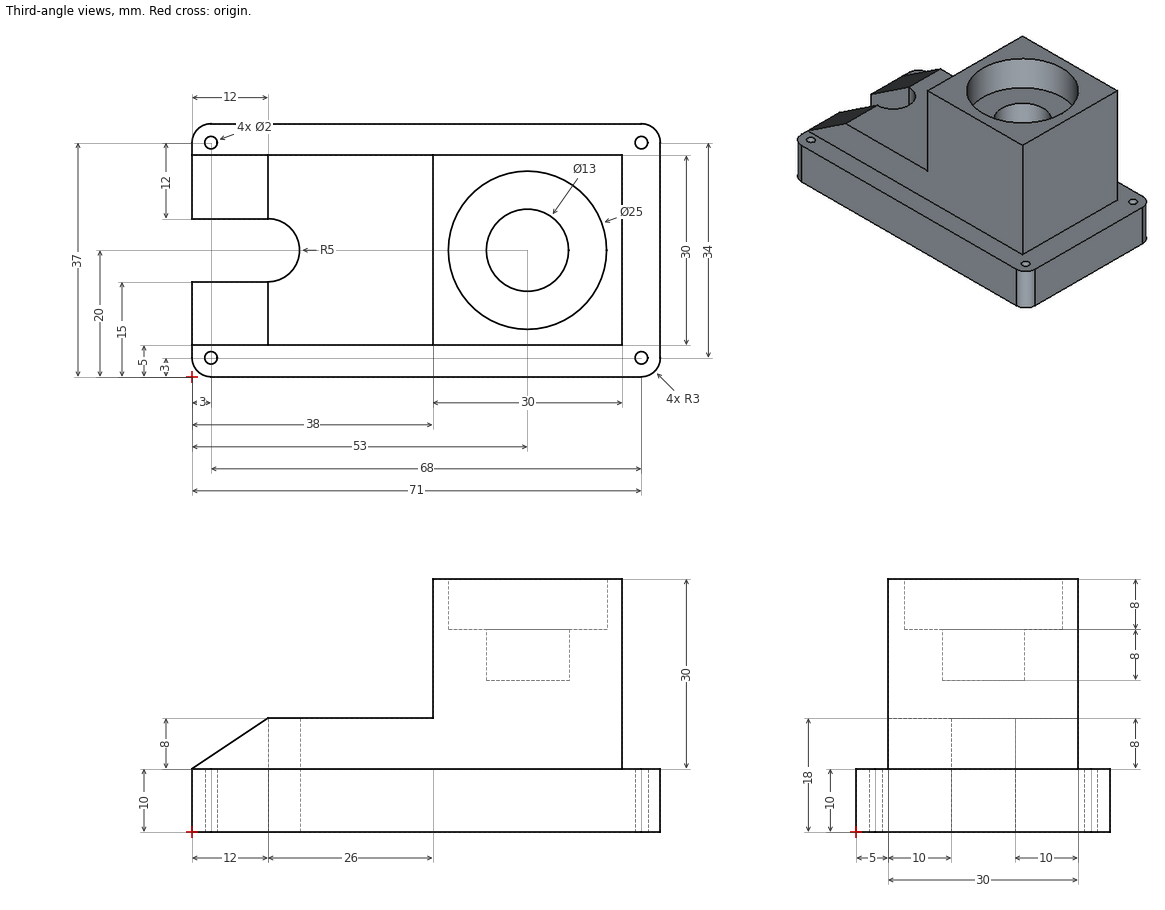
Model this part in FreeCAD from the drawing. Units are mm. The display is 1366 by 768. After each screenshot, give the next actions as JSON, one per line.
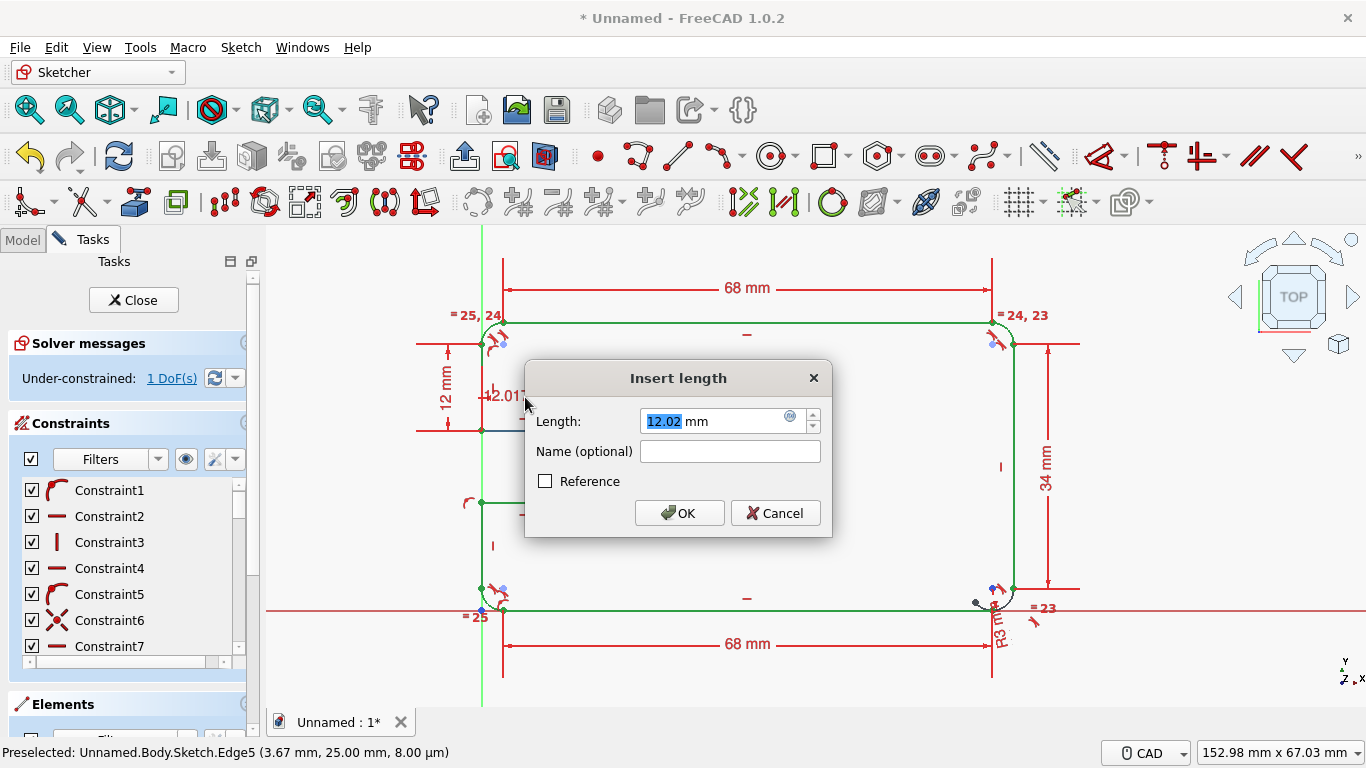
{"action": "type", "text": "12"}
{"action": "key", "text": "Return"}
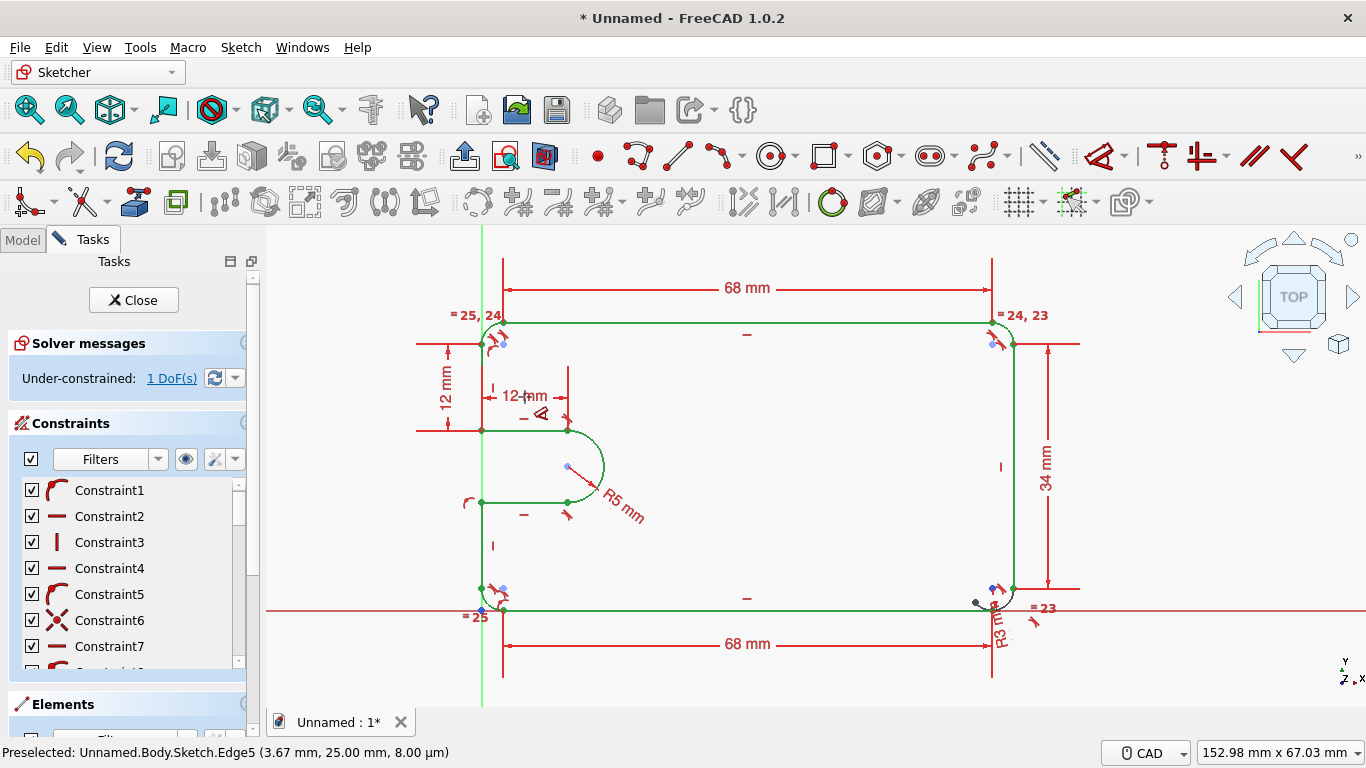
{"action": "left_click", "coordinate": [976, 603]}
{"action": "left_click", "coordinate": [615, 645]}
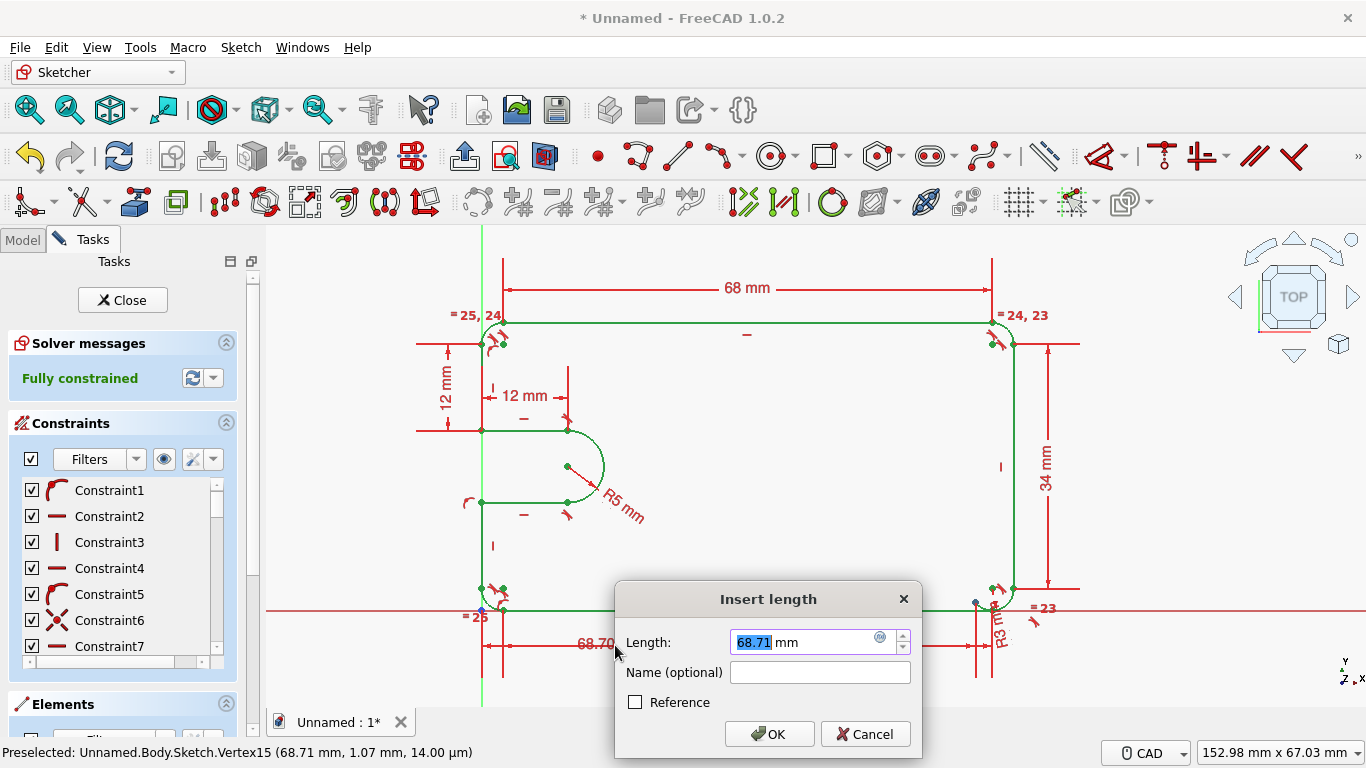
{"action": "type", "text": "71"}
{"action": "key", "text": "Return"}
{"action": "key", "text": "Escape"}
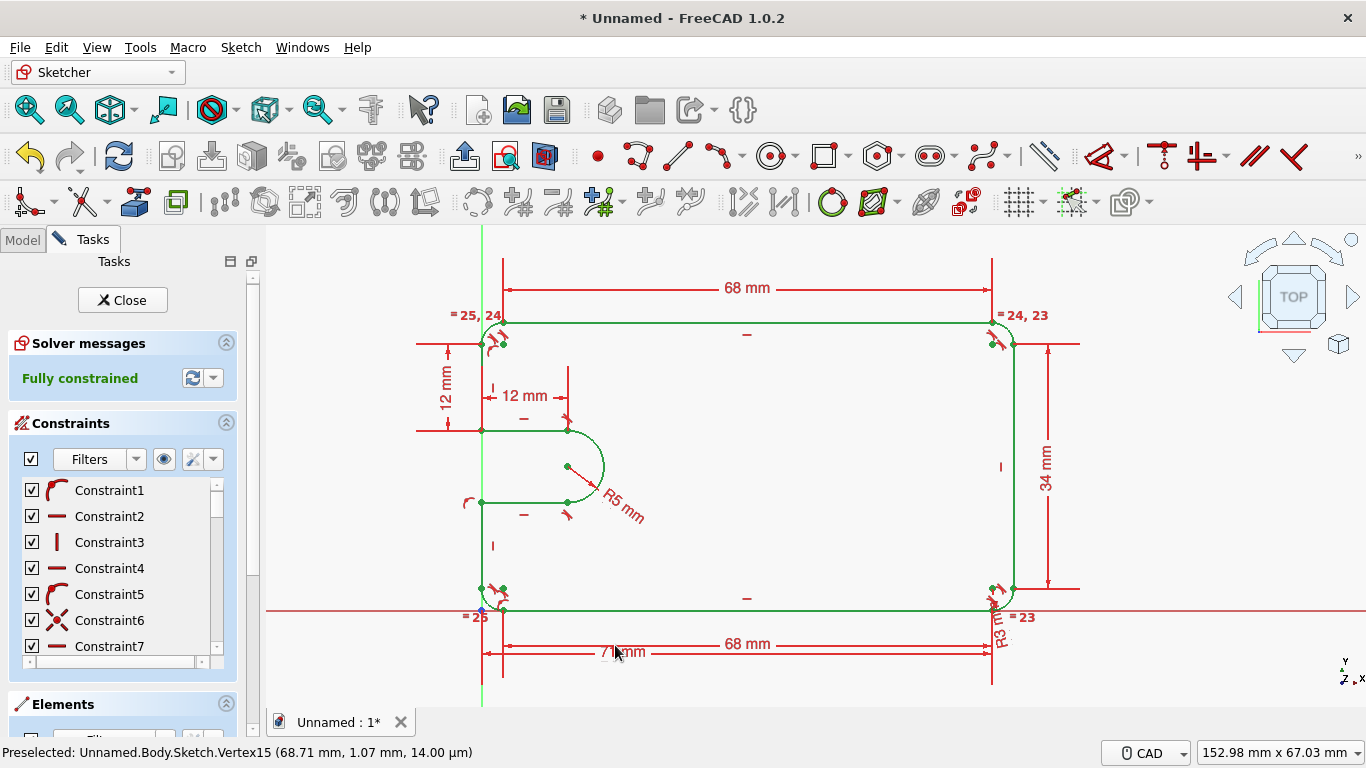
{"action": "left_click", "coordinate": [123, 300]}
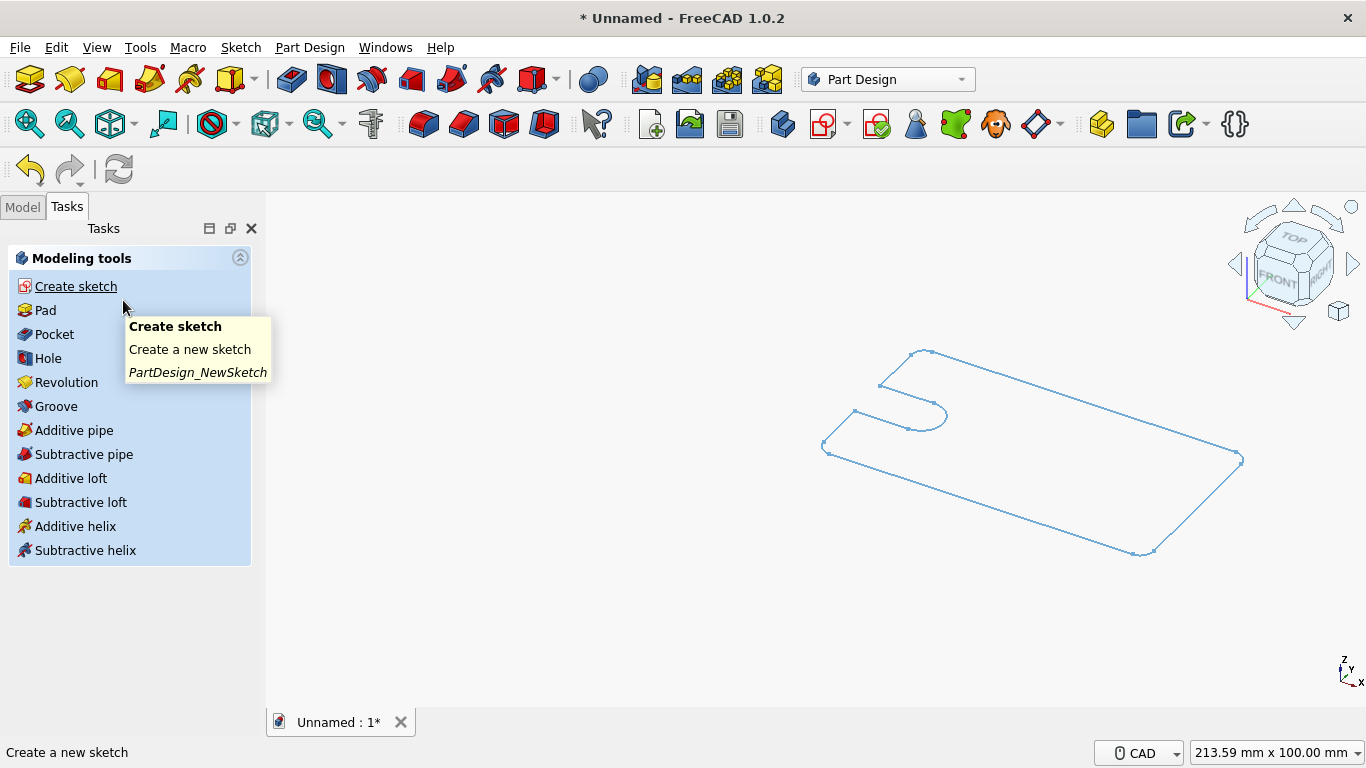
{"action": "left_click", "coordinate": [30, 80]}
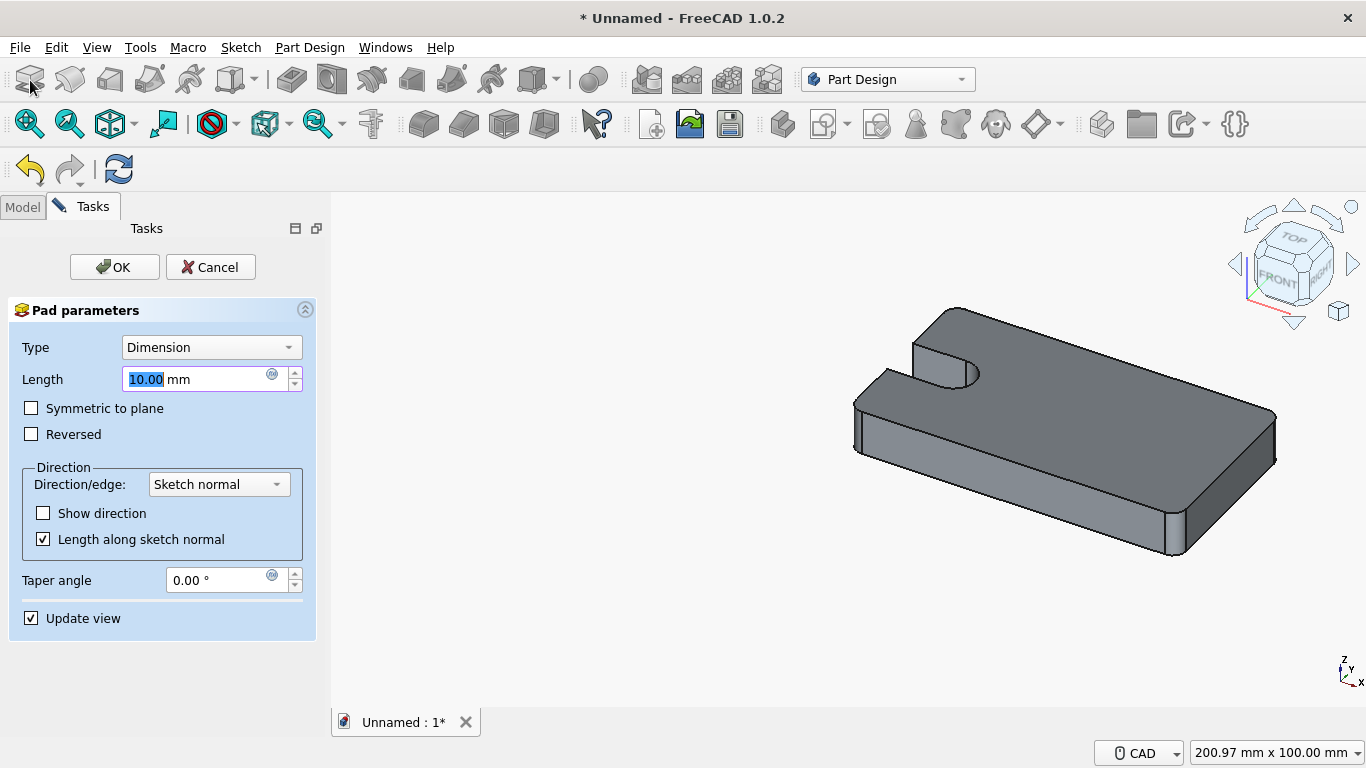
{"action": "type", "text": "10"}
{"action": "key", "text": "Tab"}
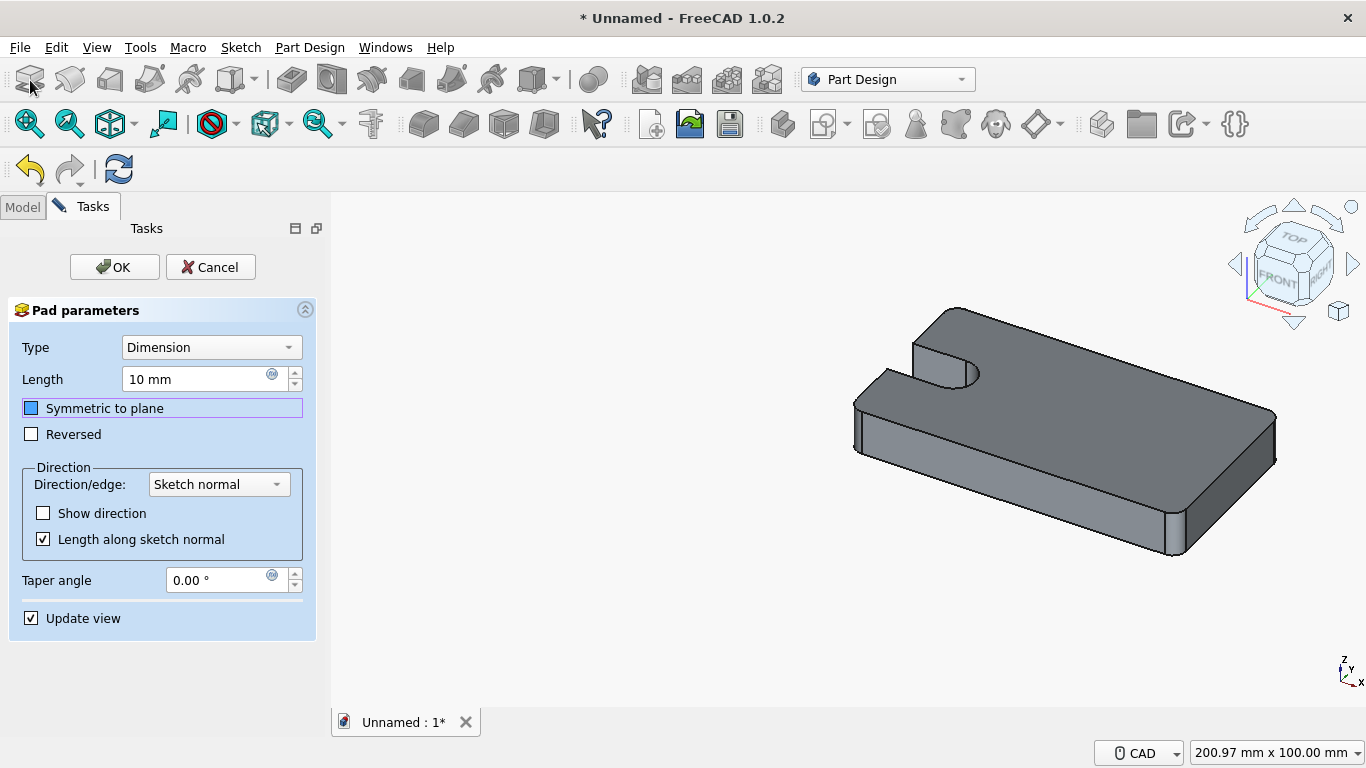
{"action": "left_click", "coordinate": [115, 267]}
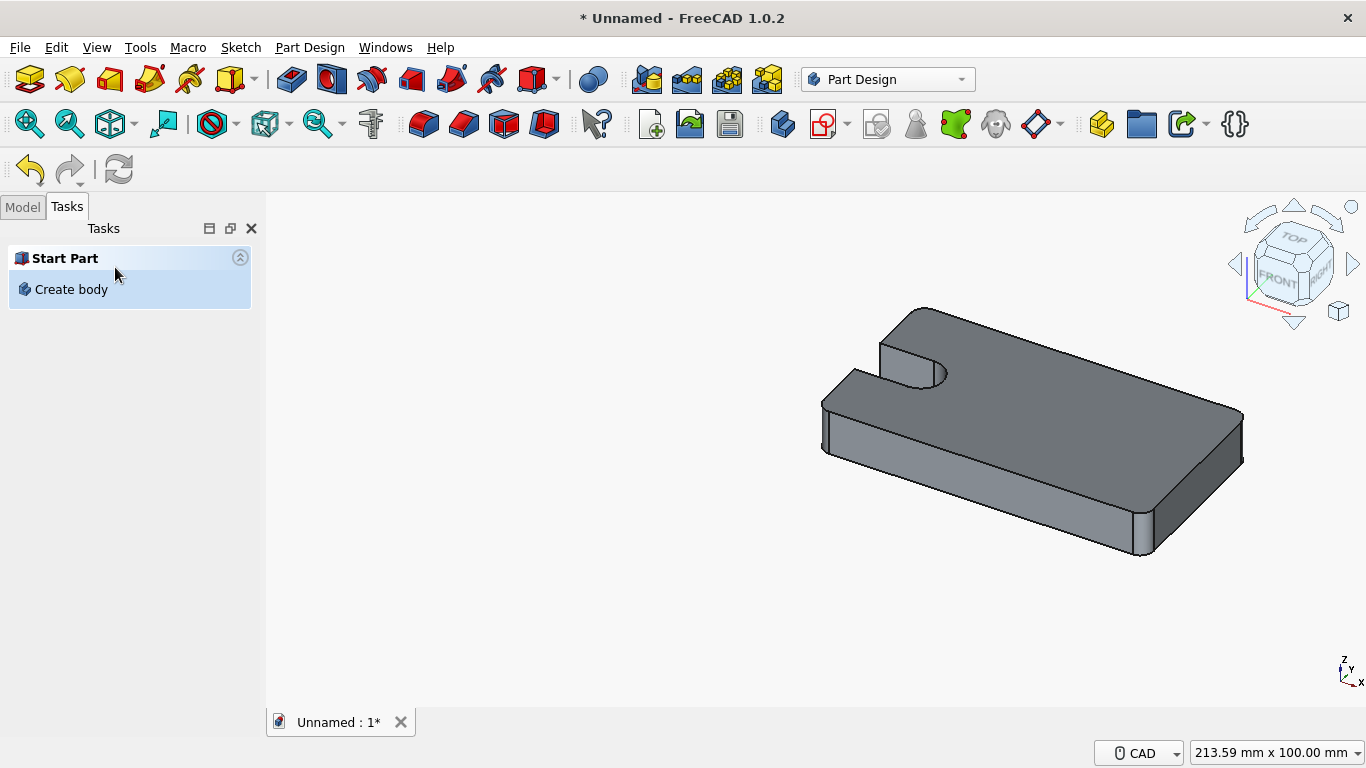
{"action": "left_click", "coordinate": [1080, 425]}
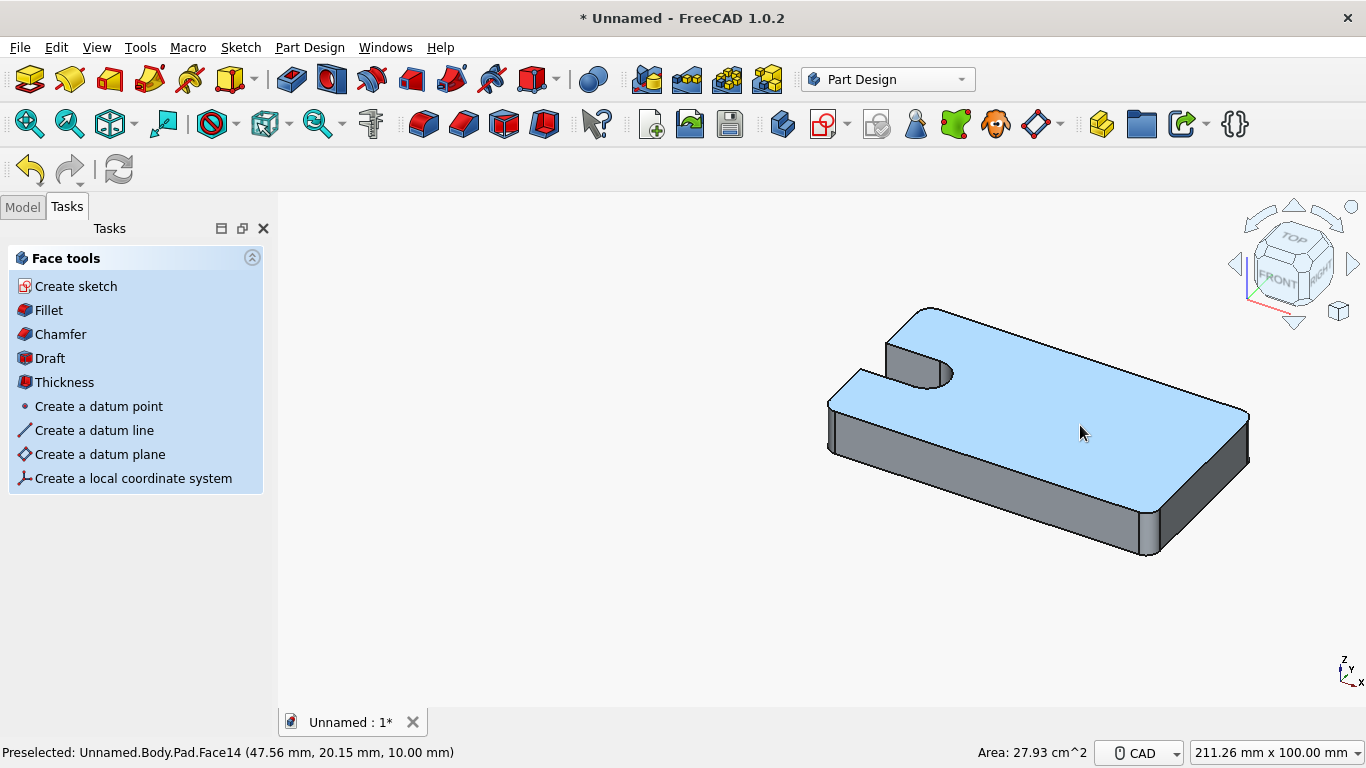
{"action": "left_click", "coordinate": [824, 124]}